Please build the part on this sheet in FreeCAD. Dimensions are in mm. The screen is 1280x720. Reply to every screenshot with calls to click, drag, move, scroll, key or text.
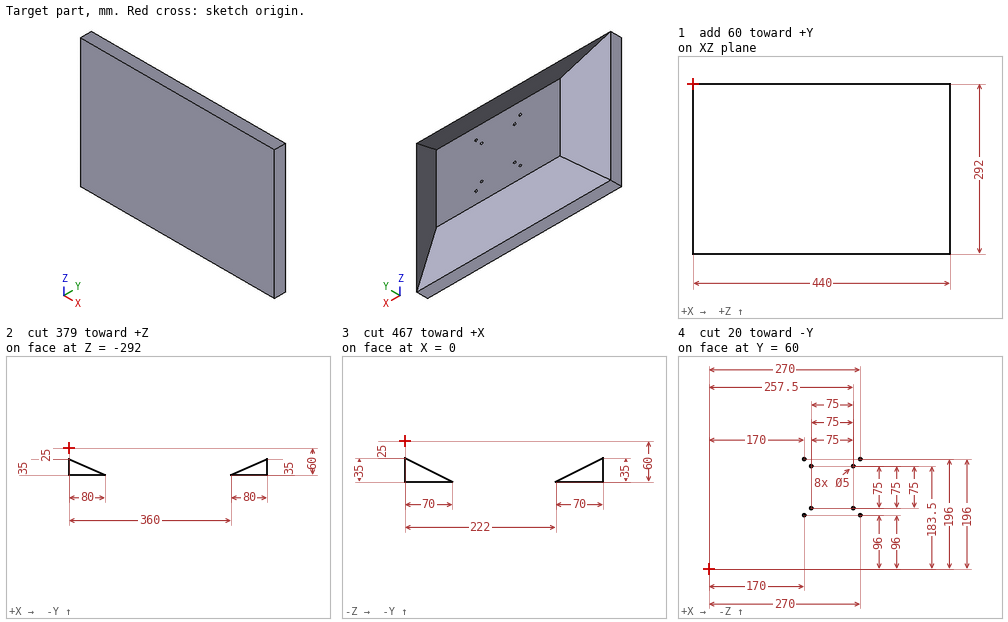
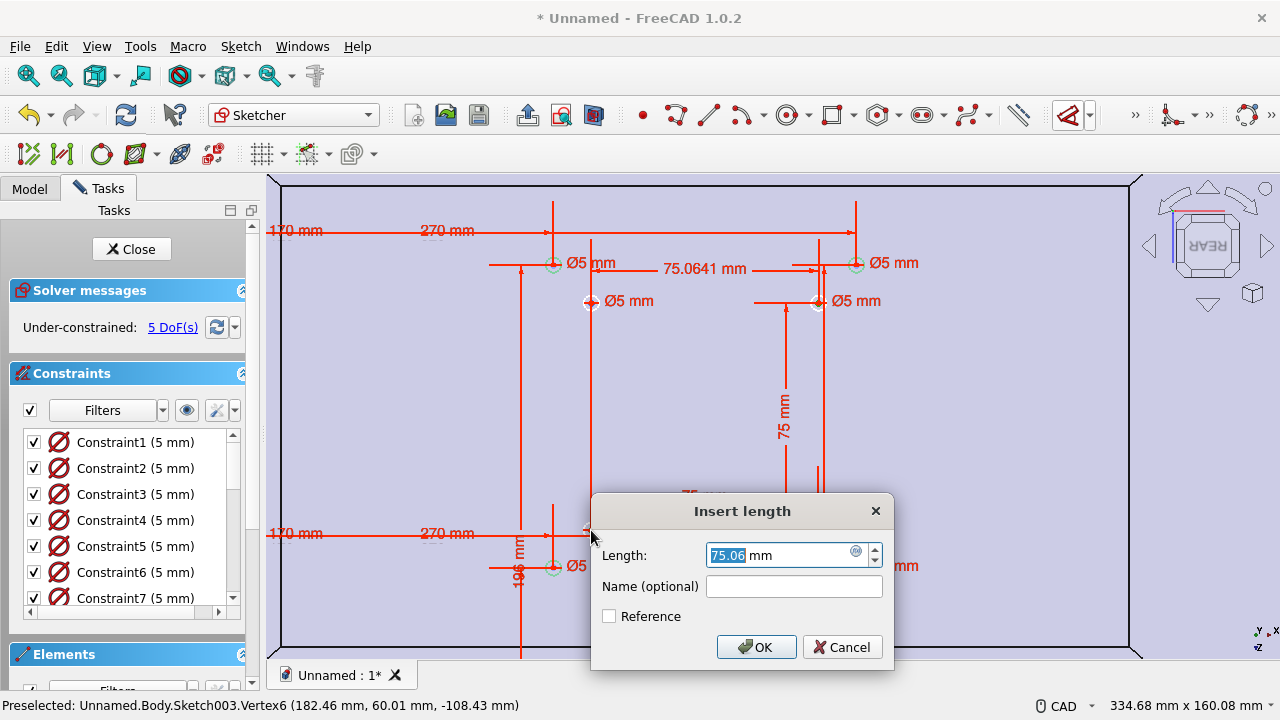
text(75)
key(Return)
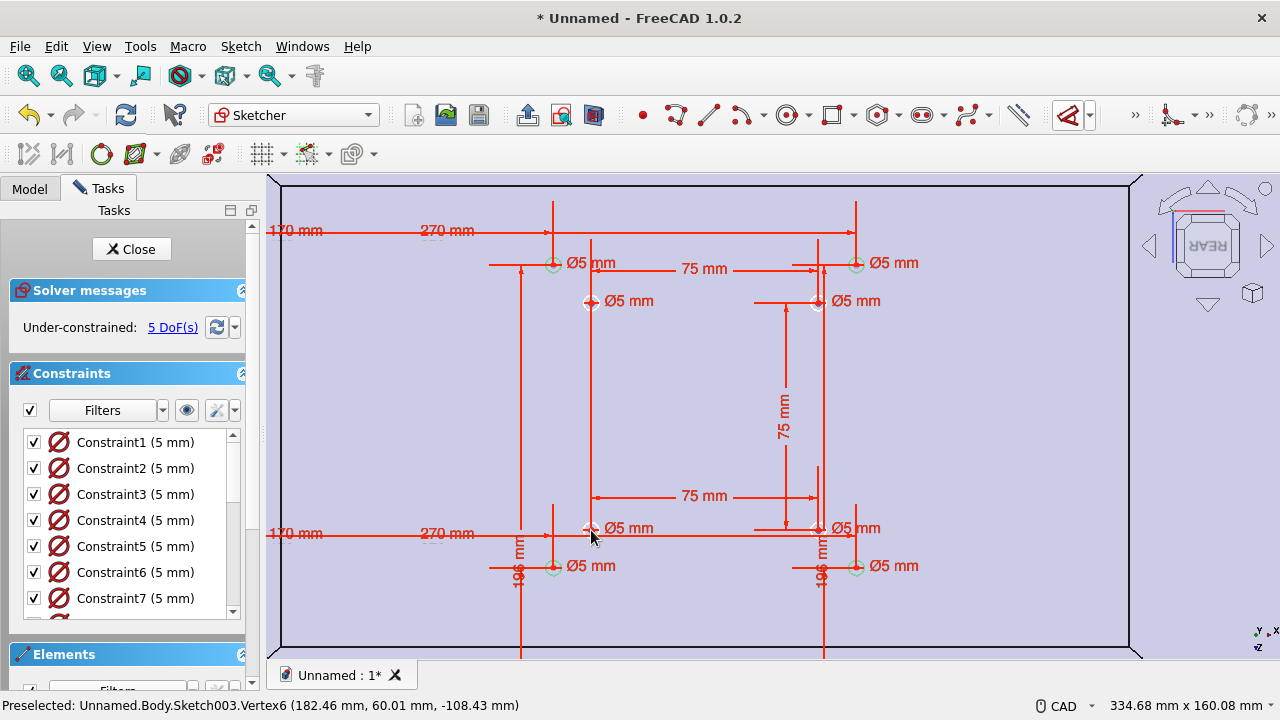
click(818, 303)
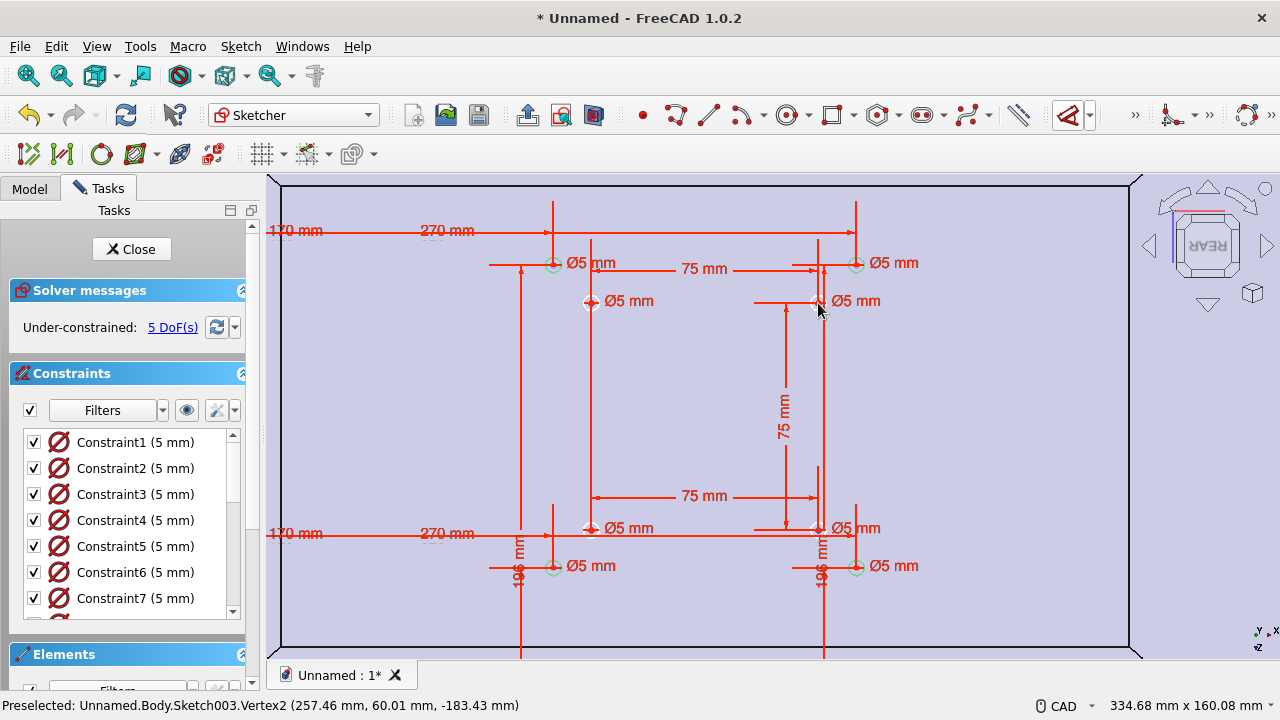
click(591, 530)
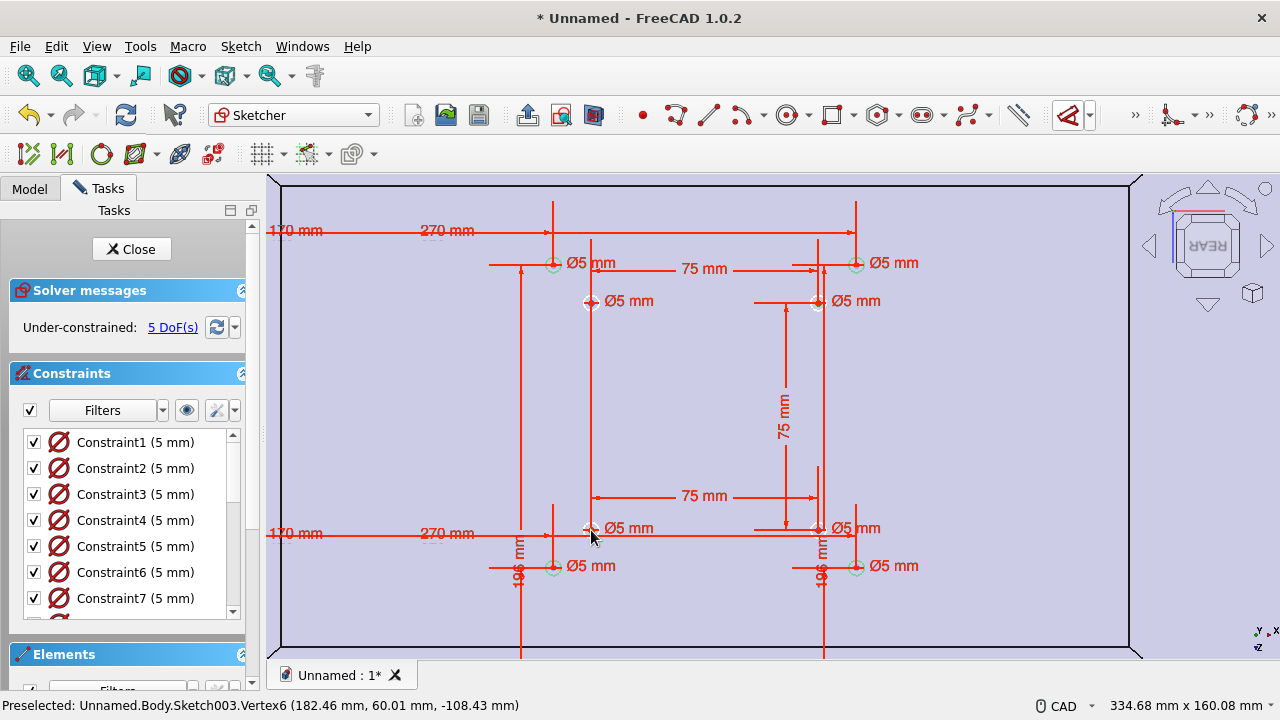
key(i)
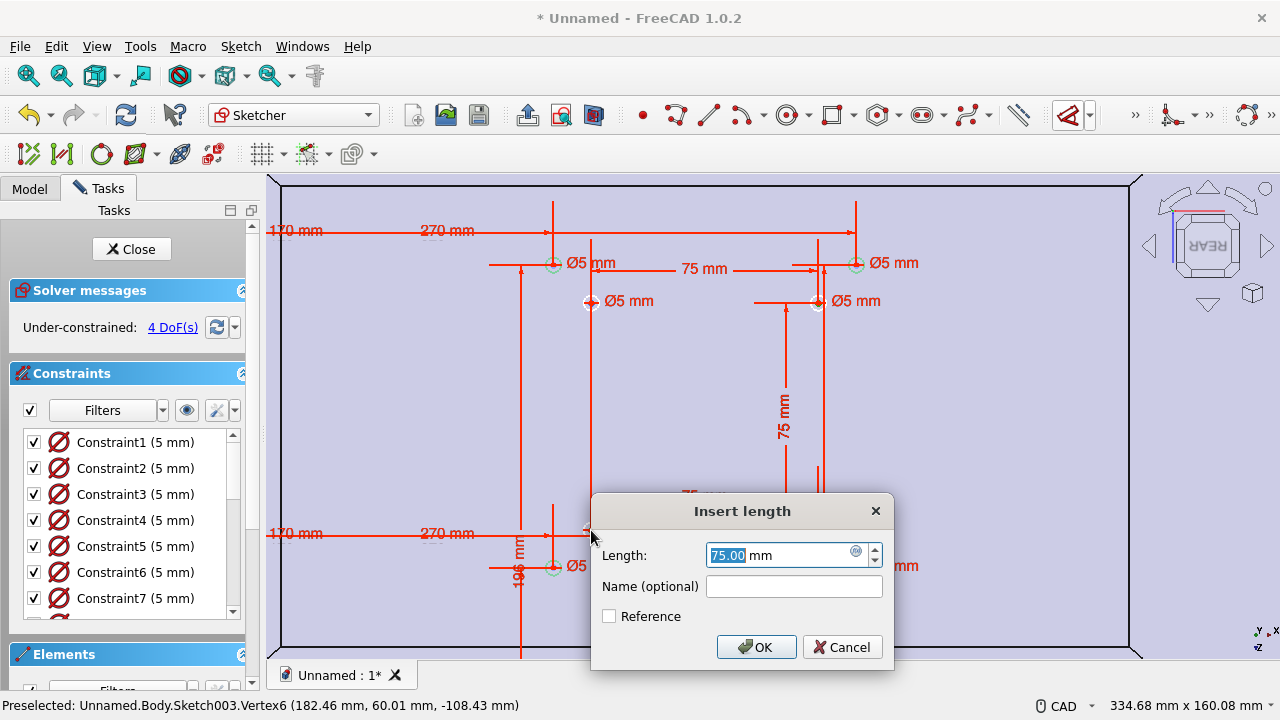
text(75)
key(Return)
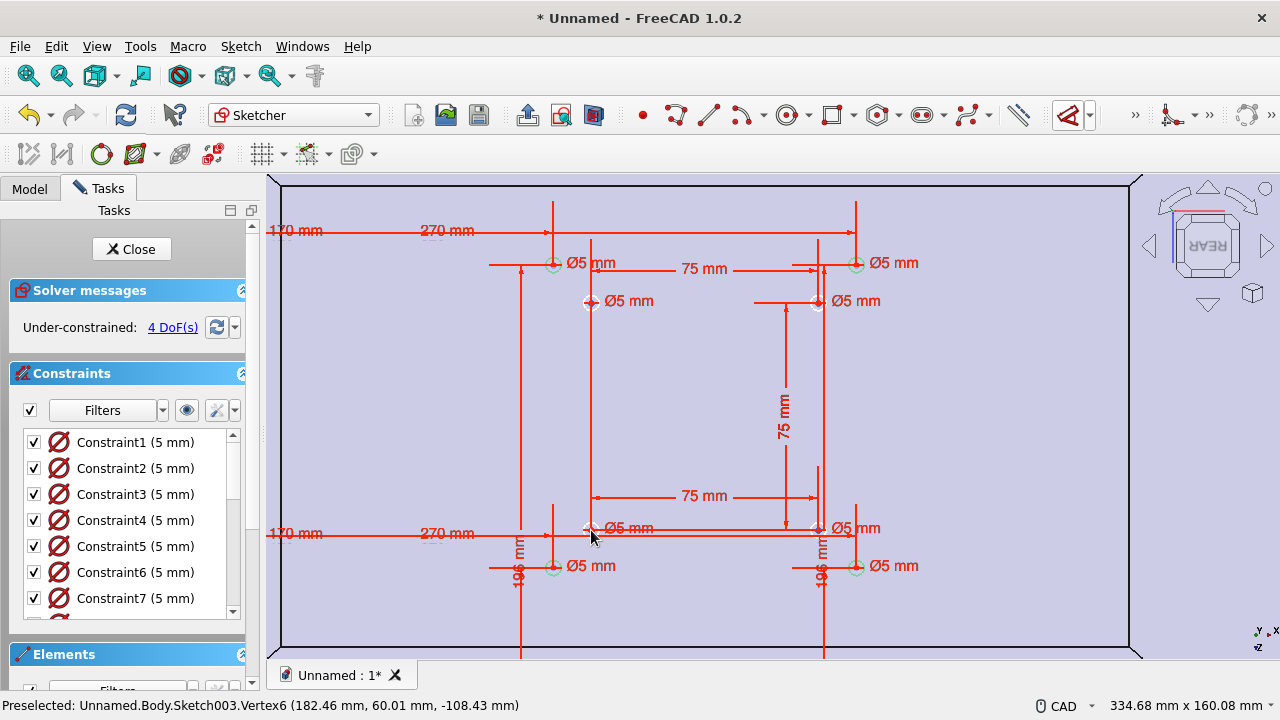
click(818, 303)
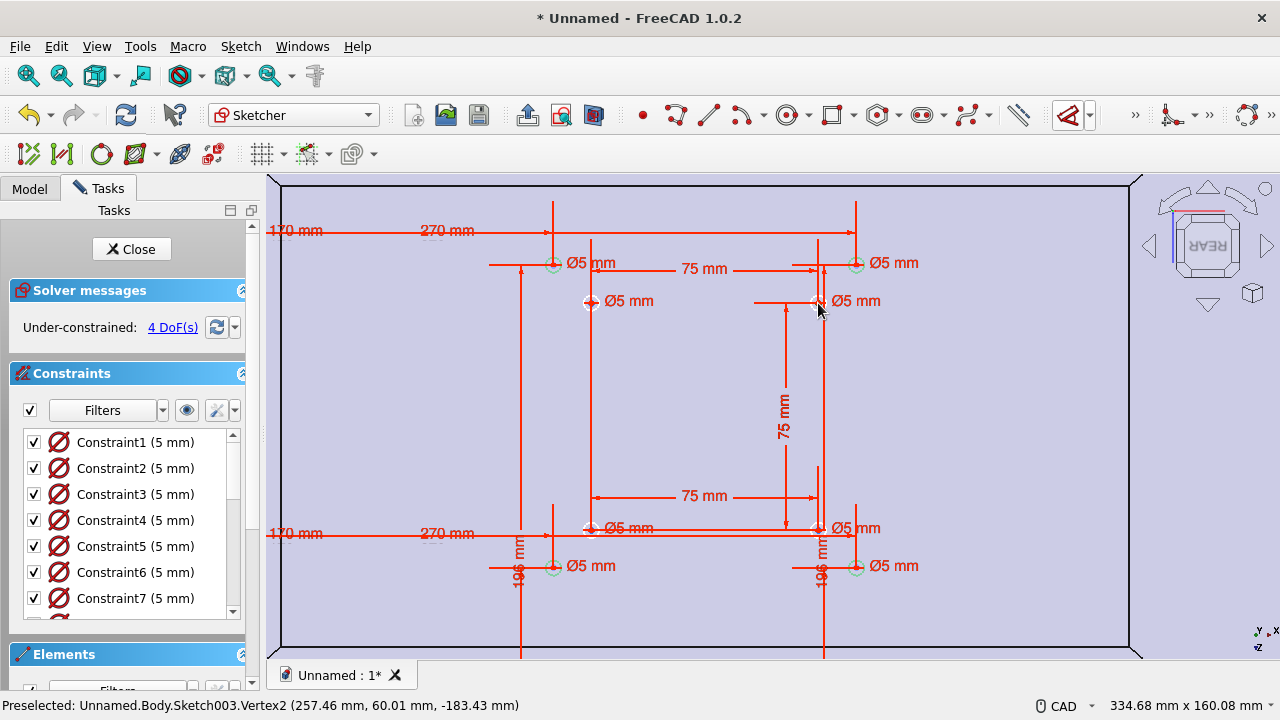
click(591, 303)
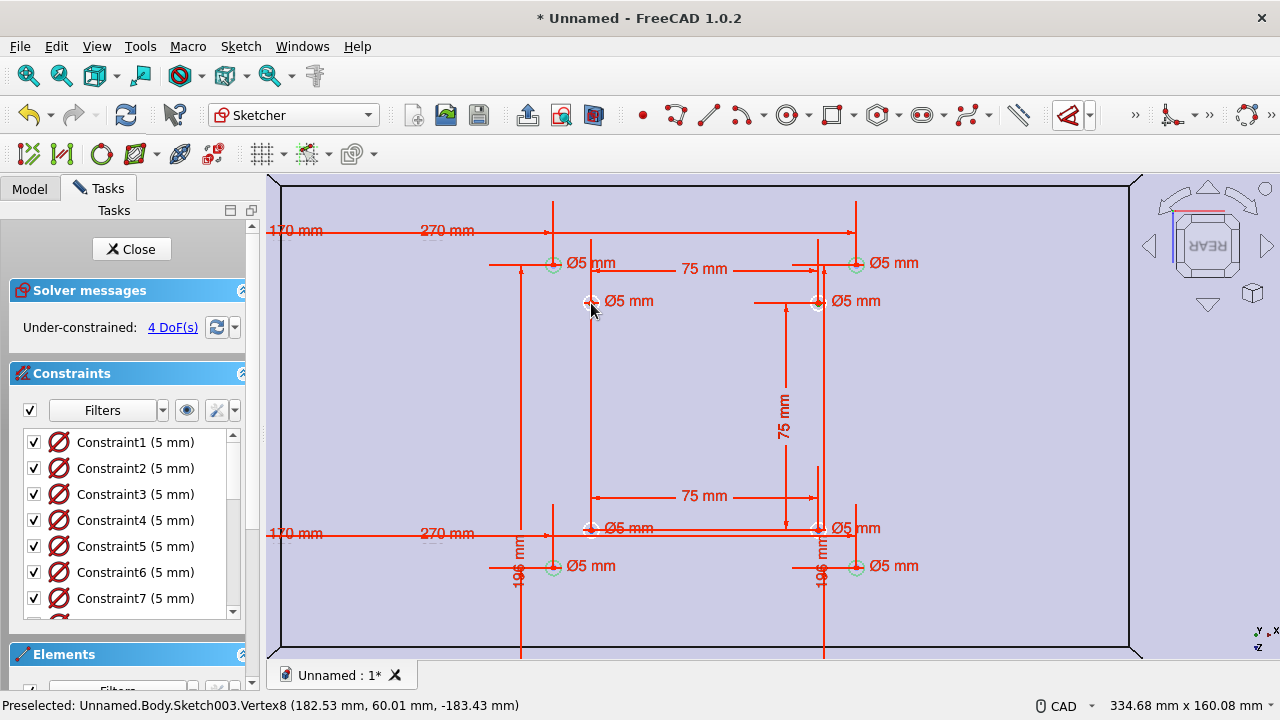
key(l)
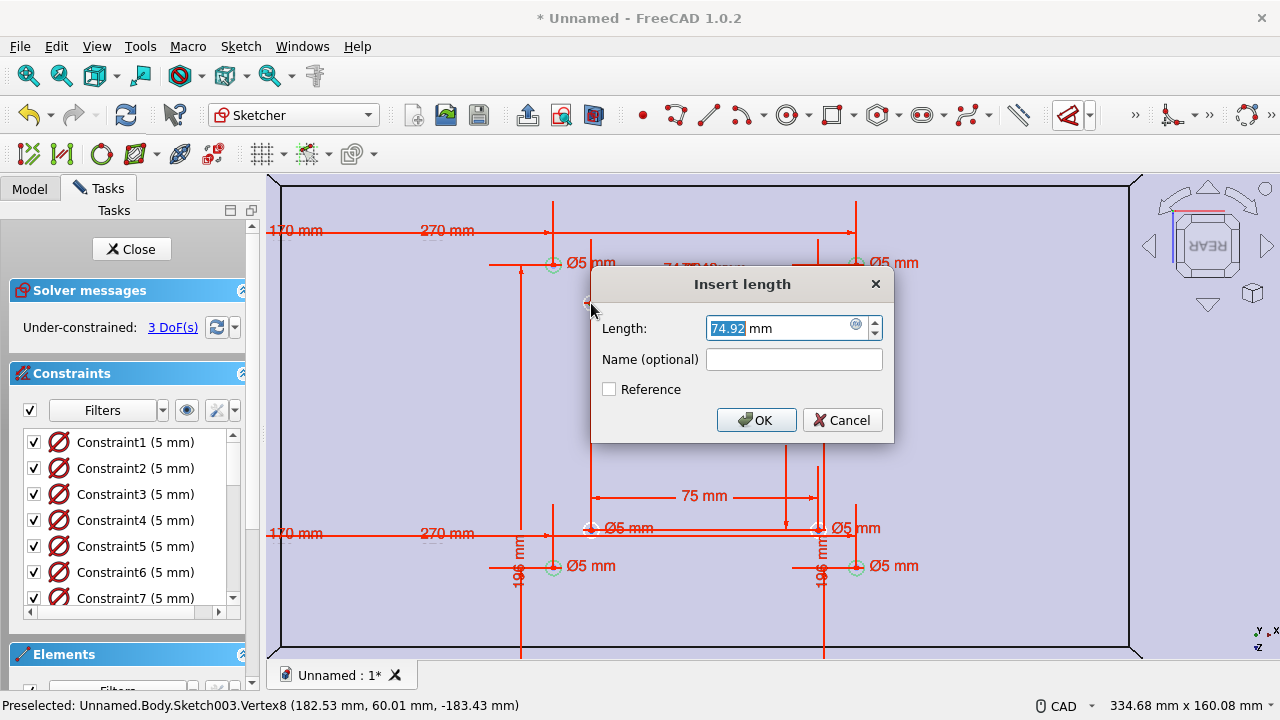
text(75)
key(Return)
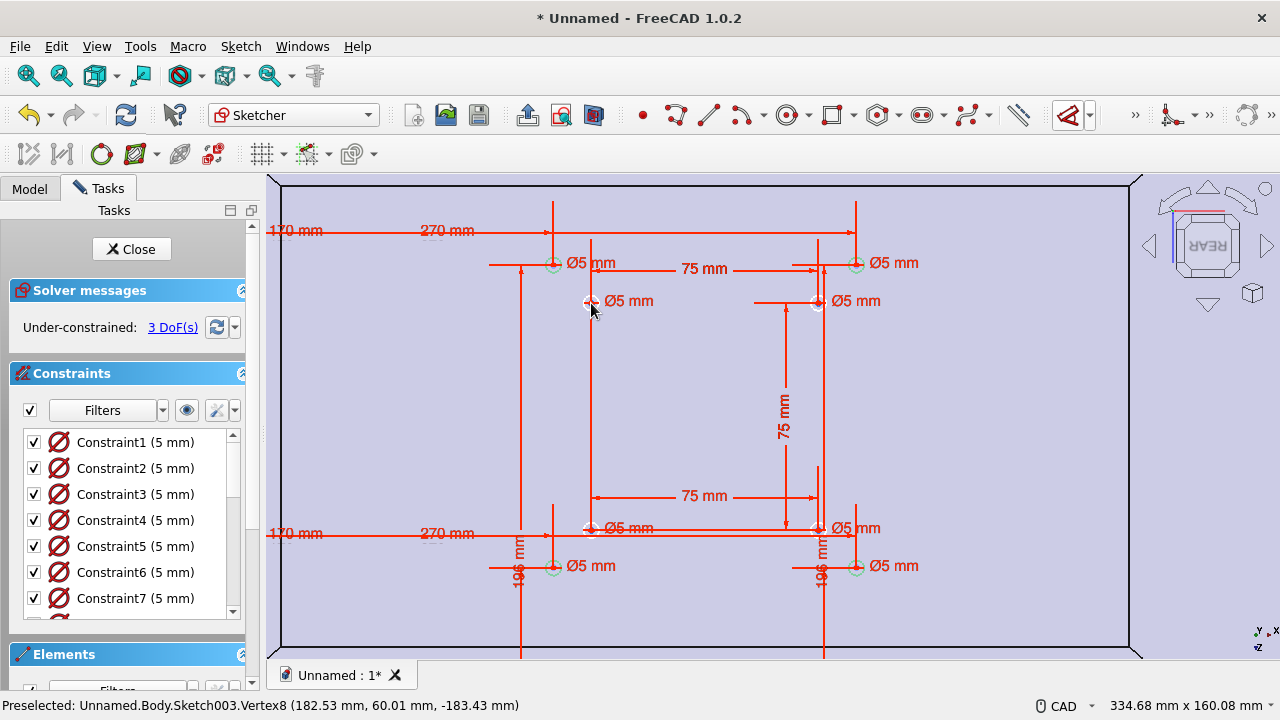
click(591, 530)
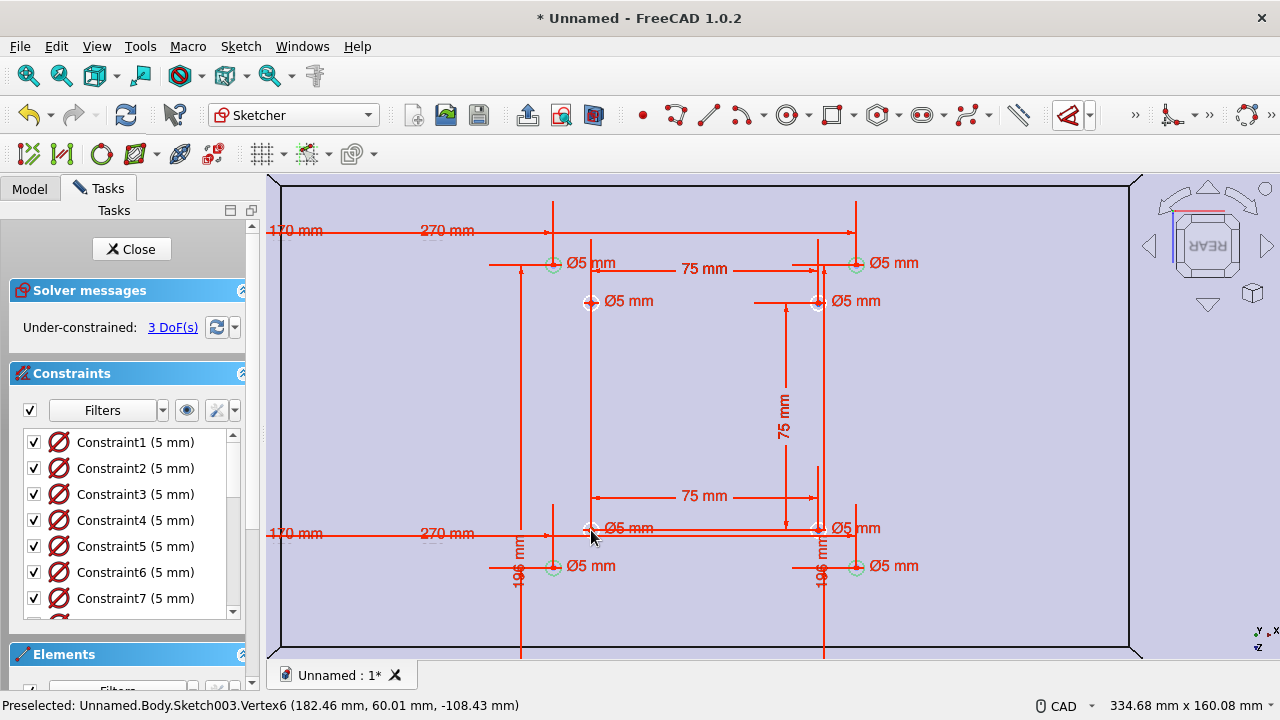
click(591, 303)